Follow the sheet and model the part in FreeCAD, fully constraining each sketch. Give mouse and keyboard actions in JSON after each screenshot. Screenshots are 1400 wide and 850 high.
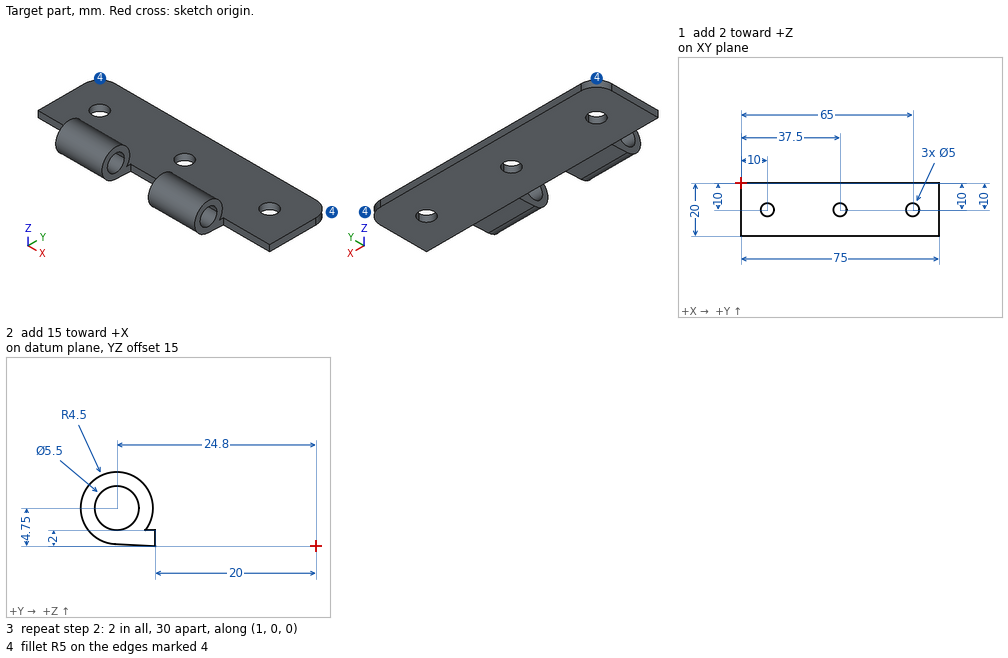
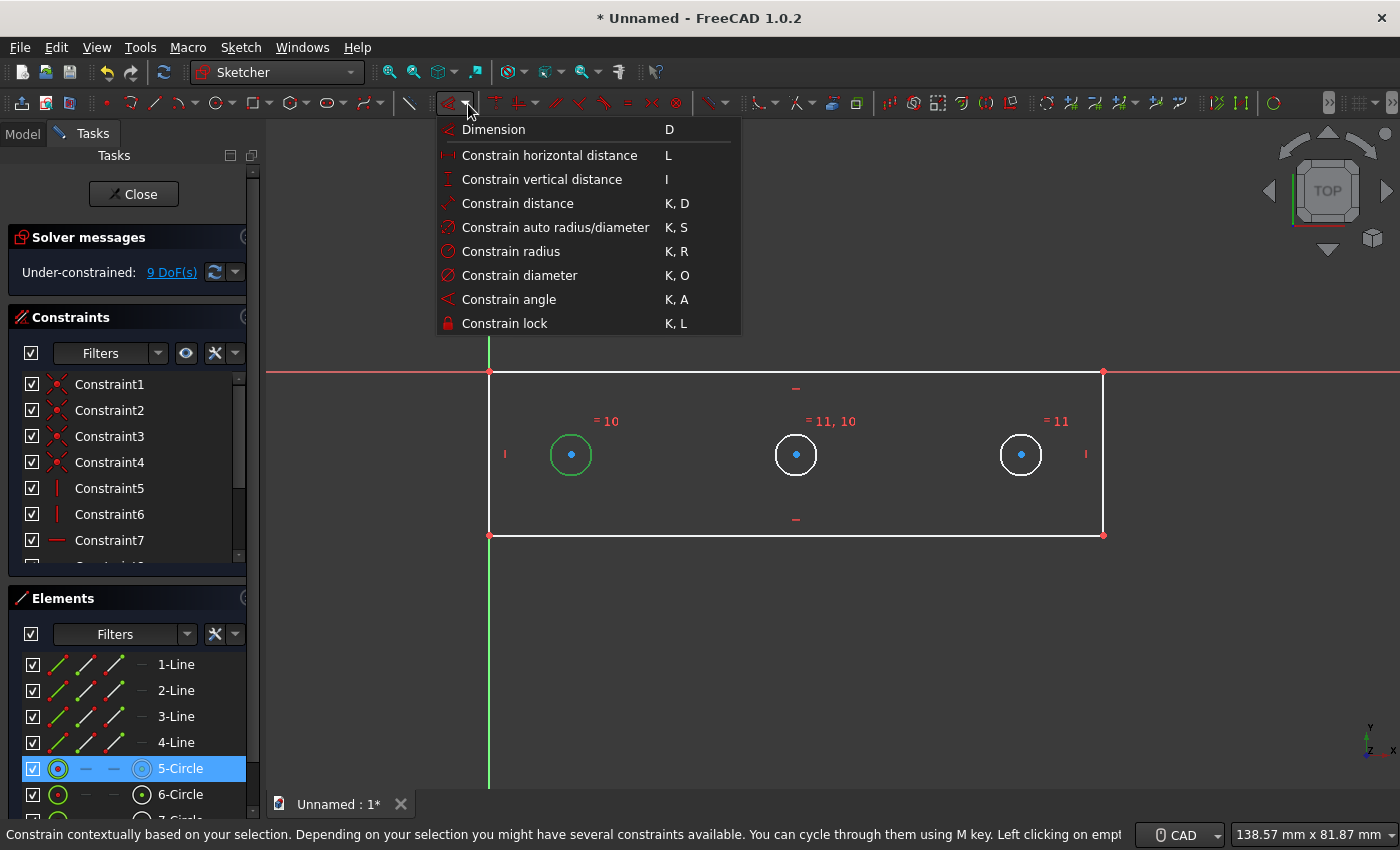
{"action": "left_click", "coordinate": [589, 275]}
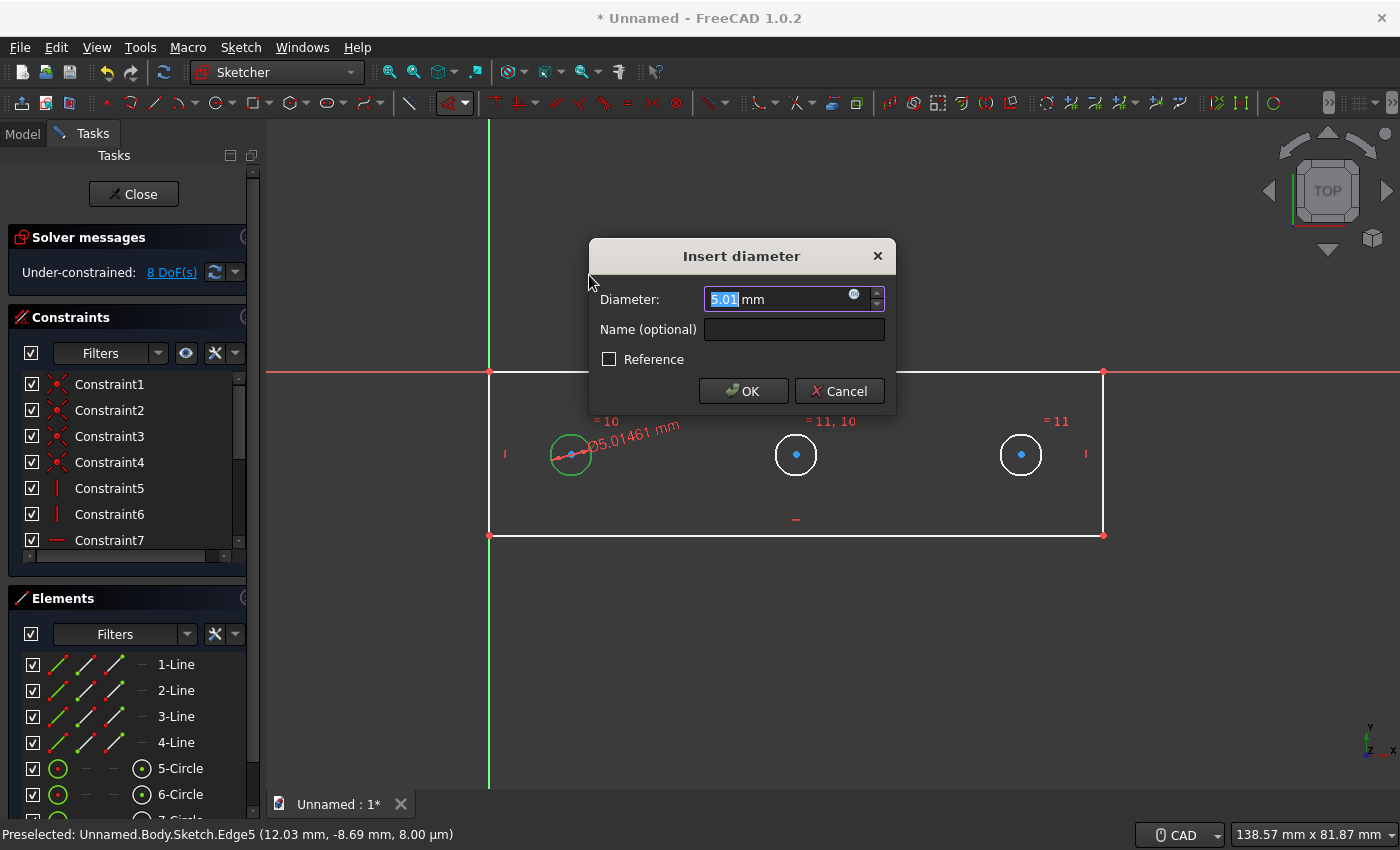
{"action": "type", "text": "5"}
{"action": "key", "text": "Return"}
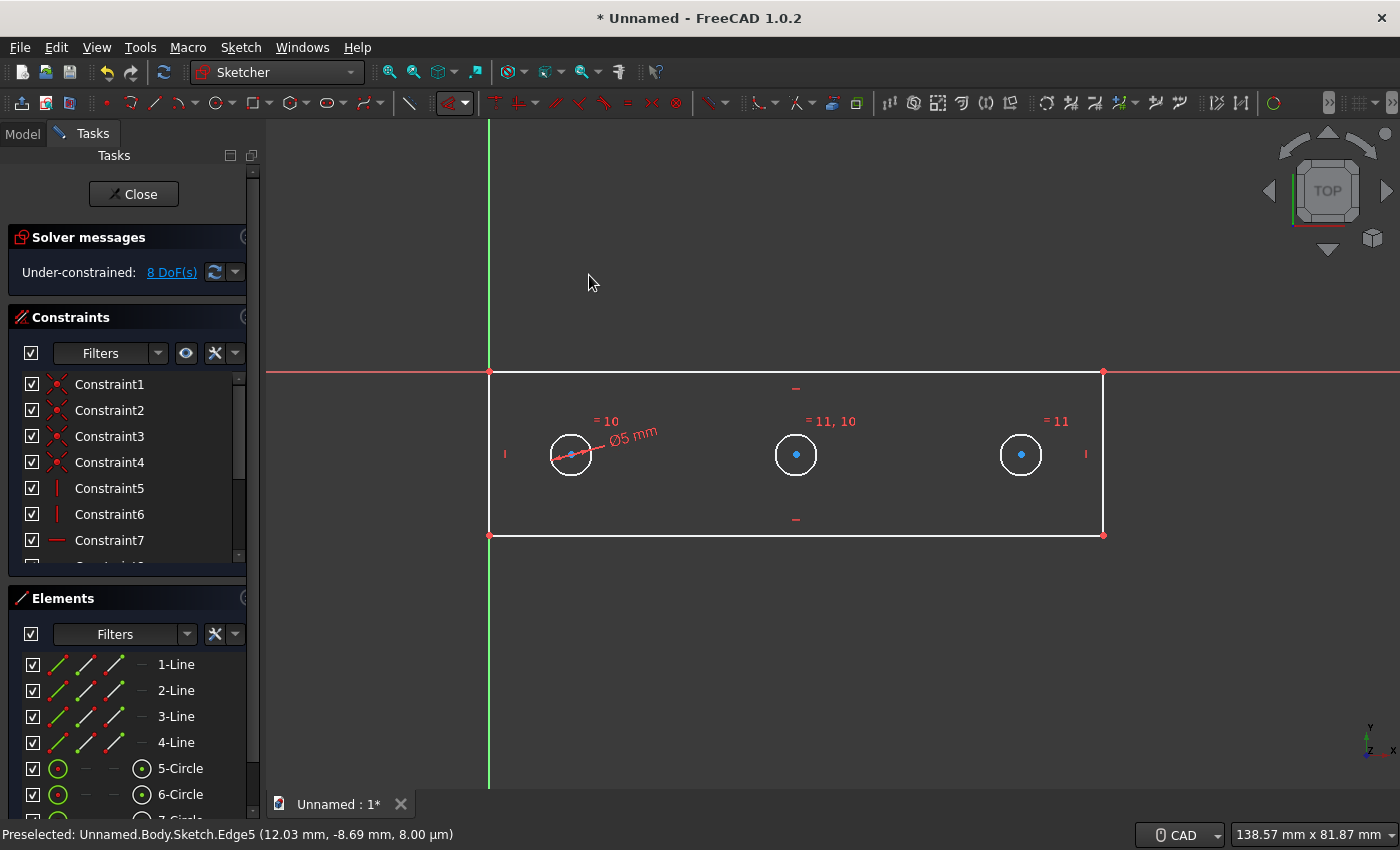
{"action": "left_click", "coordinate": [489, 421]}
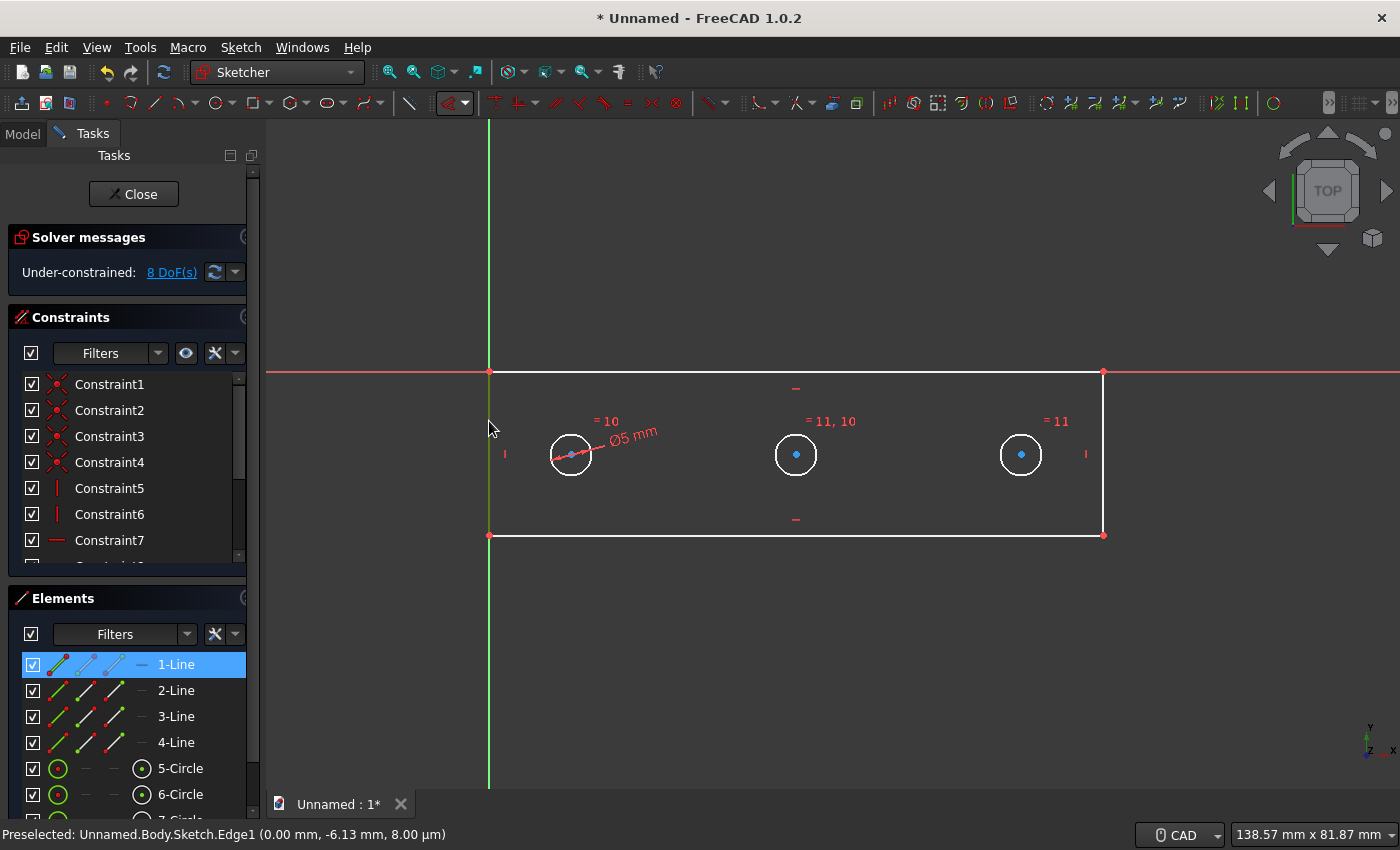
{"action": "key", "text": "i"}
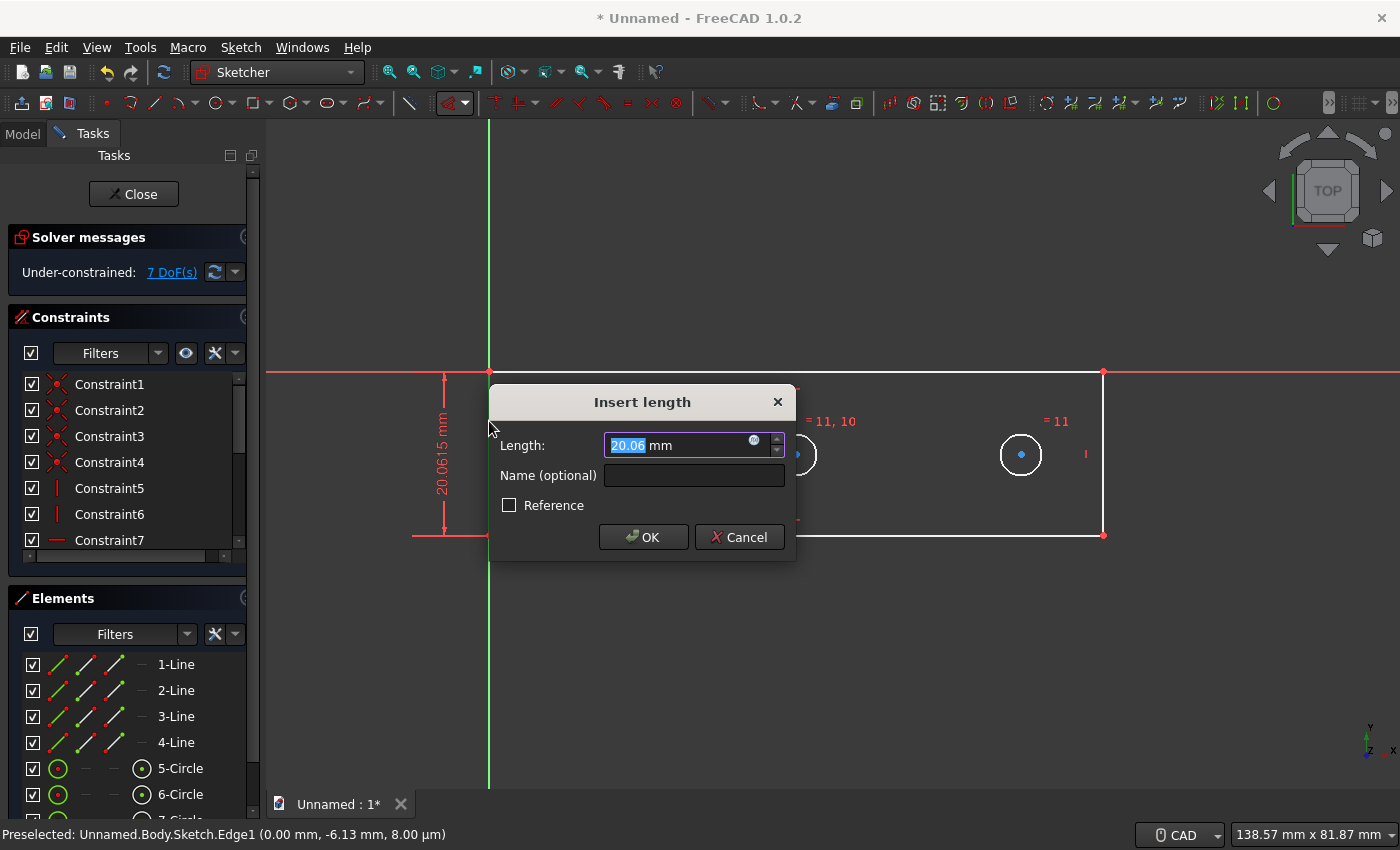
{"action": "type", "text": "20"}
{"action": "key", "text": "Return"}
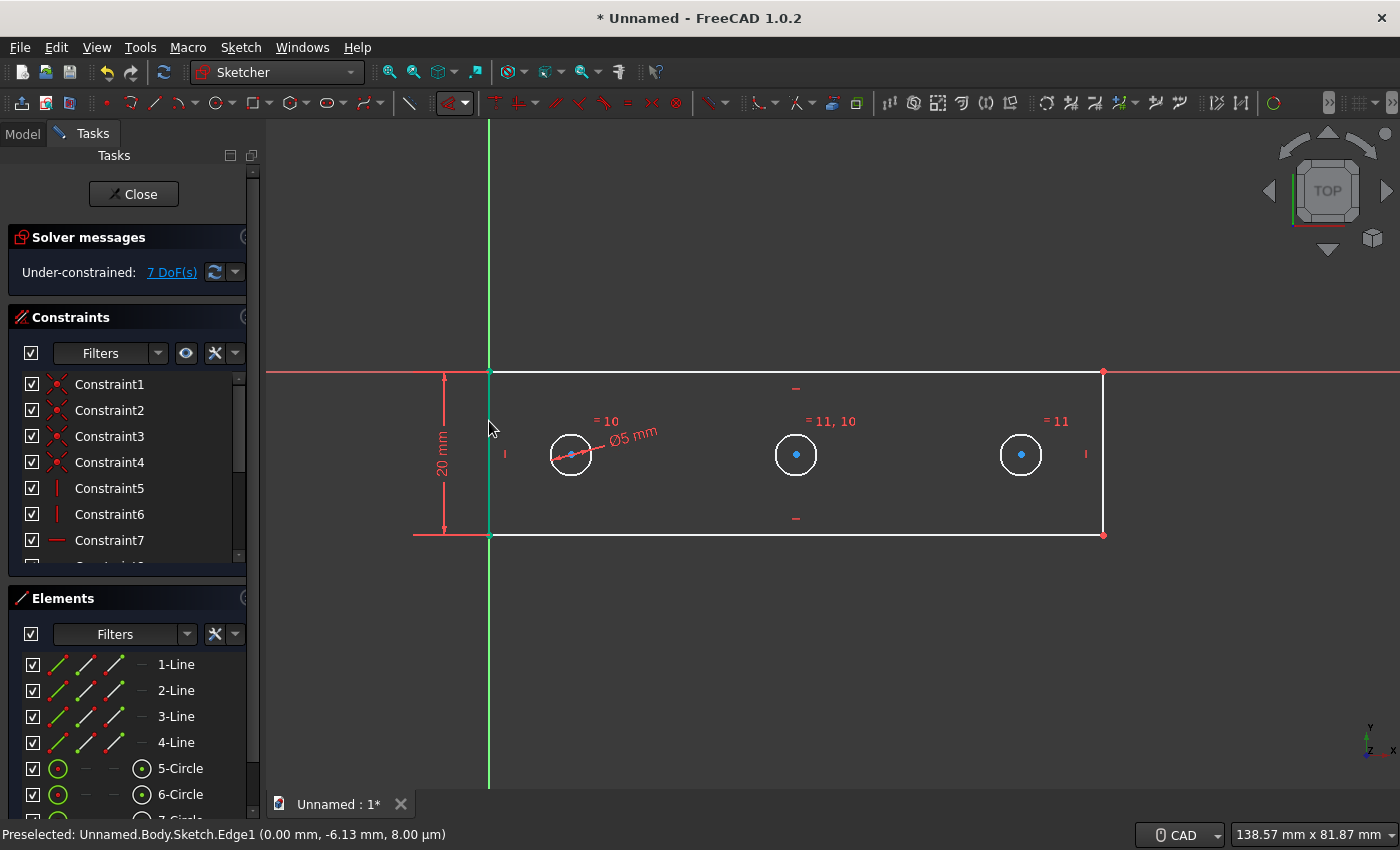
{"action": "left_click", "coordinate": [673, 535]}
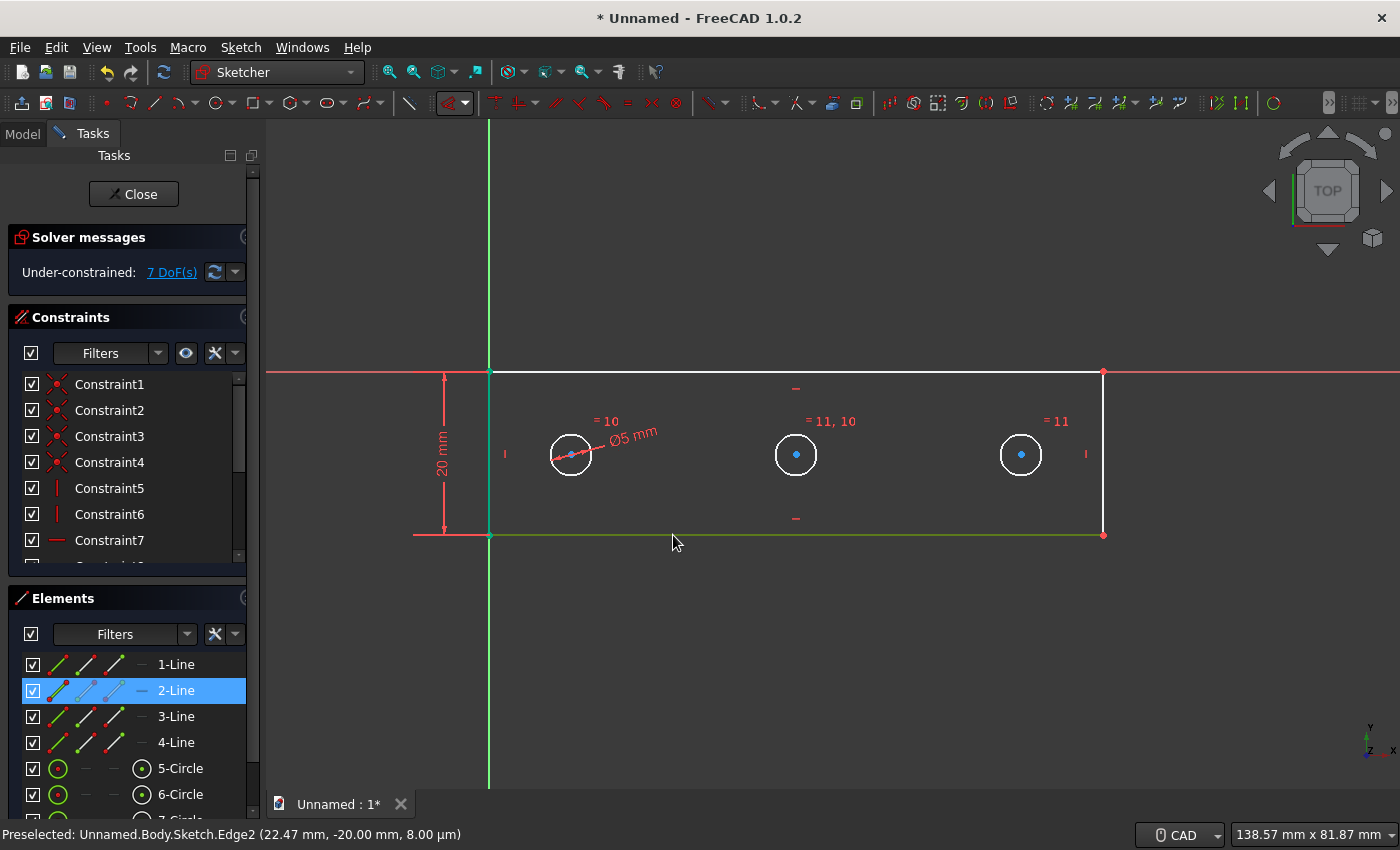
{"action": "key", "text": "l"}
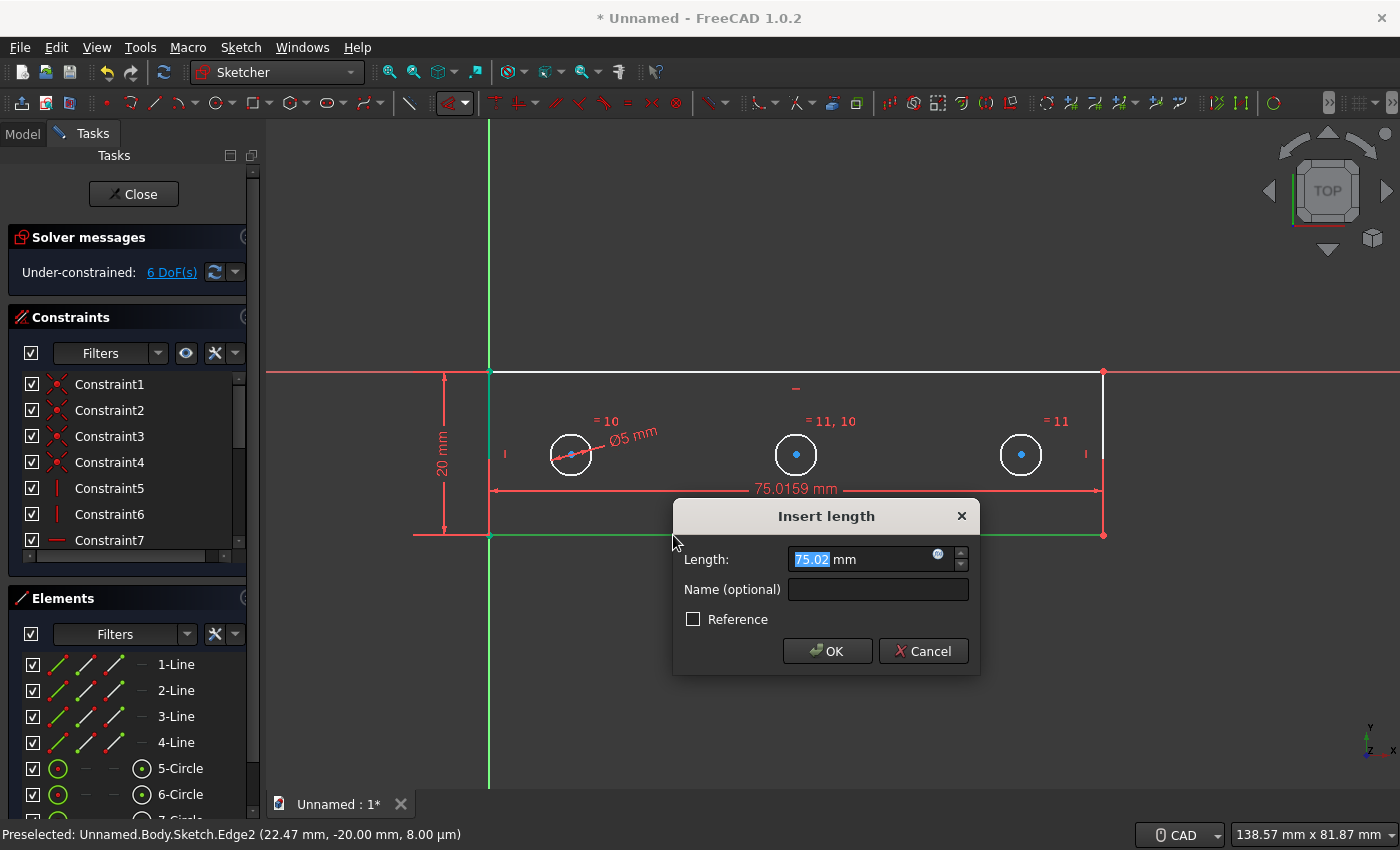
{"action": "type", "text": "75"}
{"action": "key", "text": "Return"}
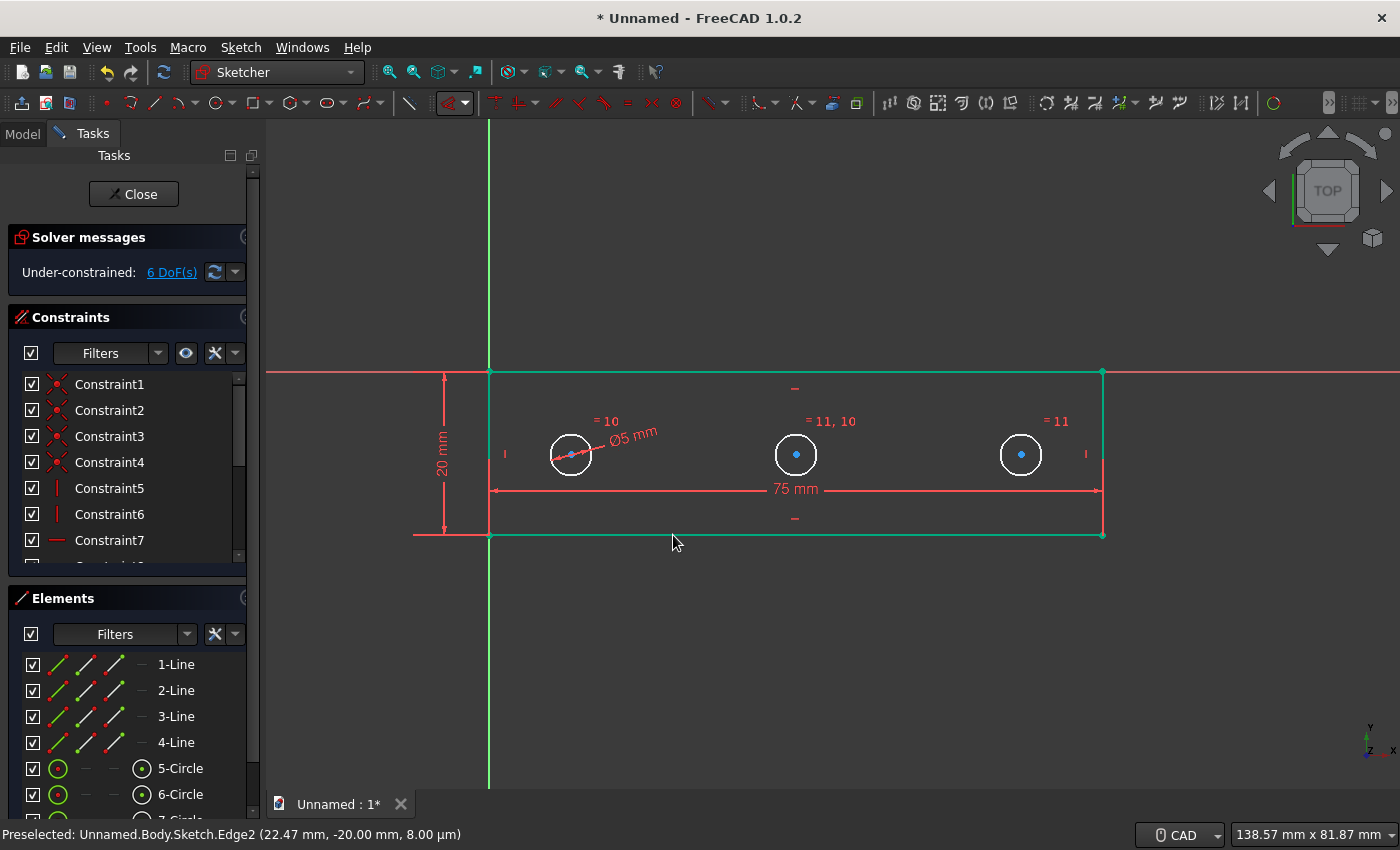
{"action": "left_click", "coordinate": [571, 455]}